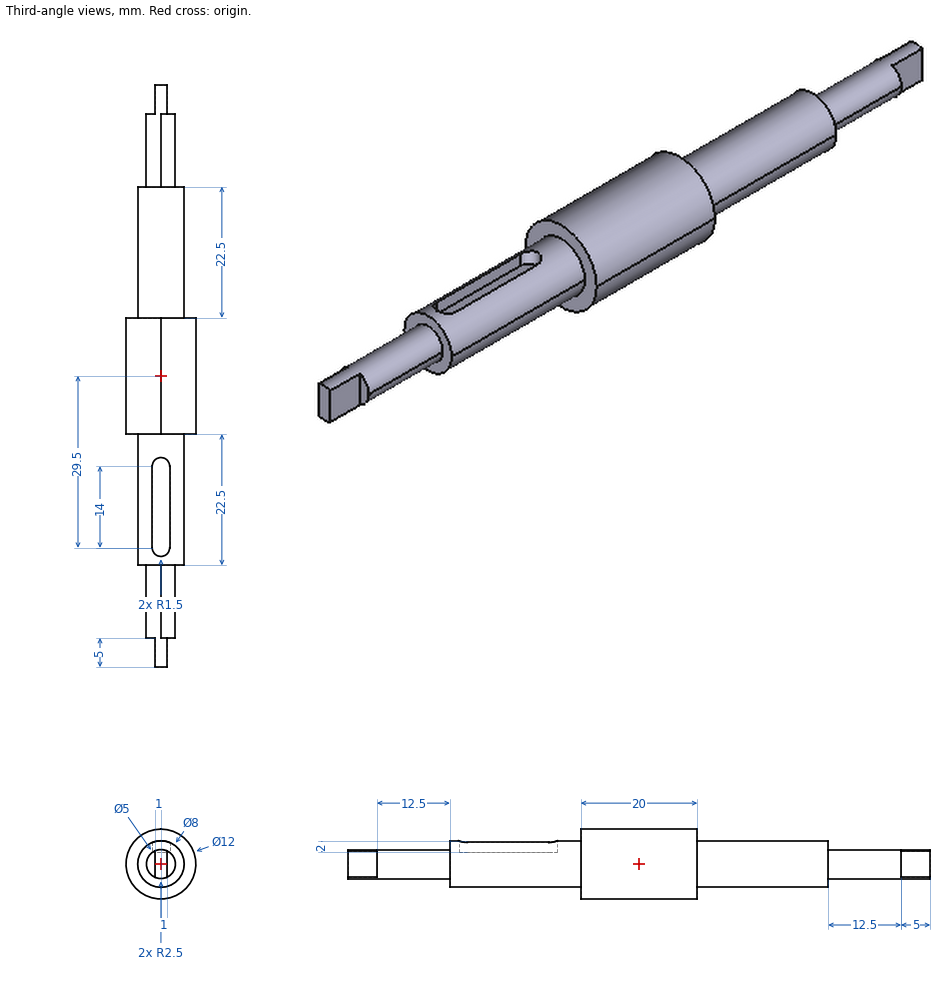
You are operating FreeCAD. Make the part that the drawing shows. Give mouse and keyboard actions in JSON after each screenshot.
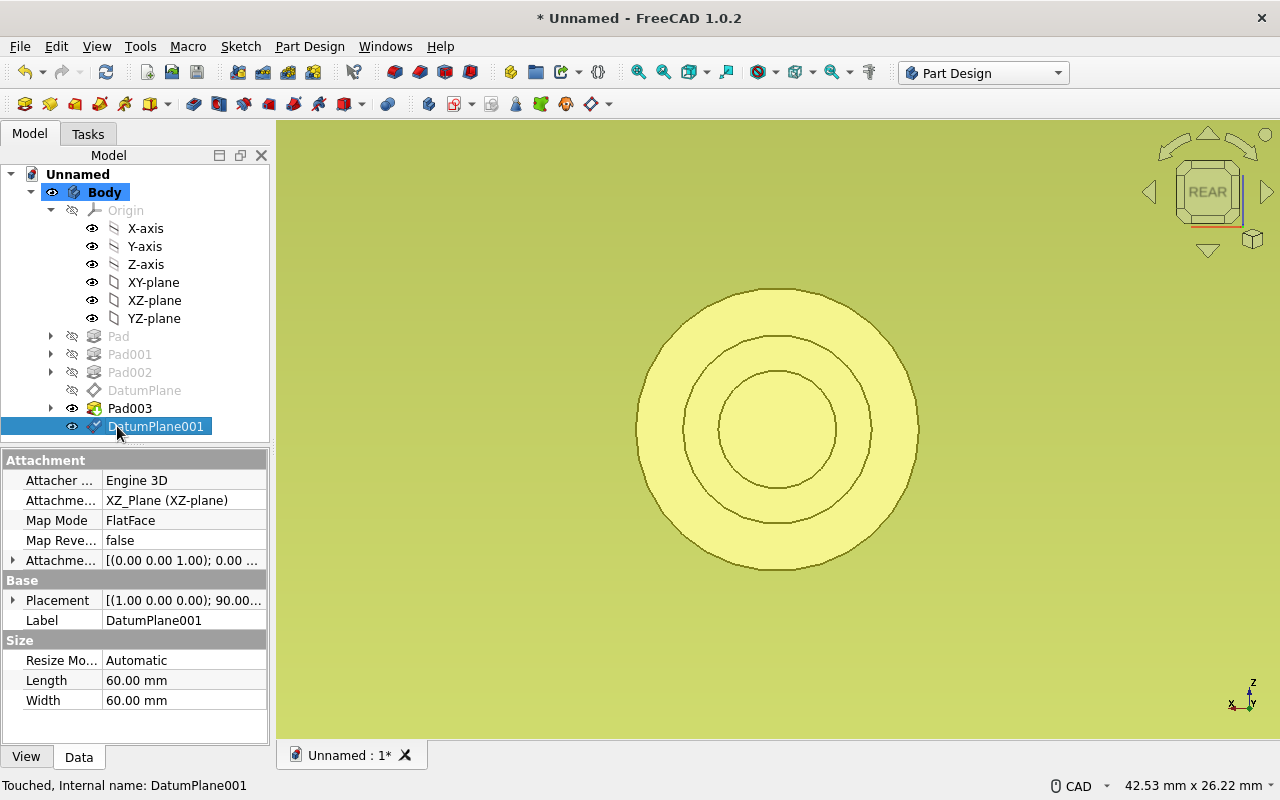
{"action": "left_click", "coordinate": [454, 104]}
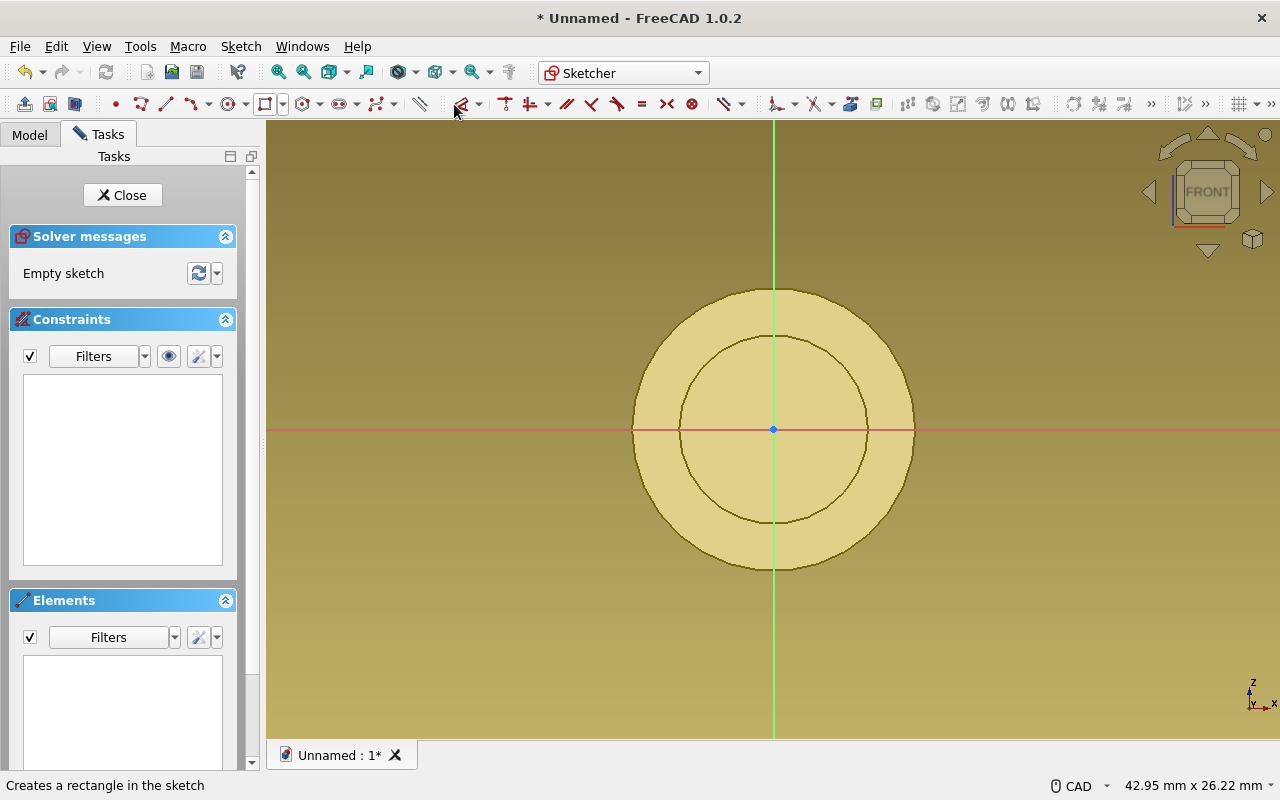
{"action": "scroll", "coordinate": [803, 429], "scroll_direction": "up", "scroll_amount": 6}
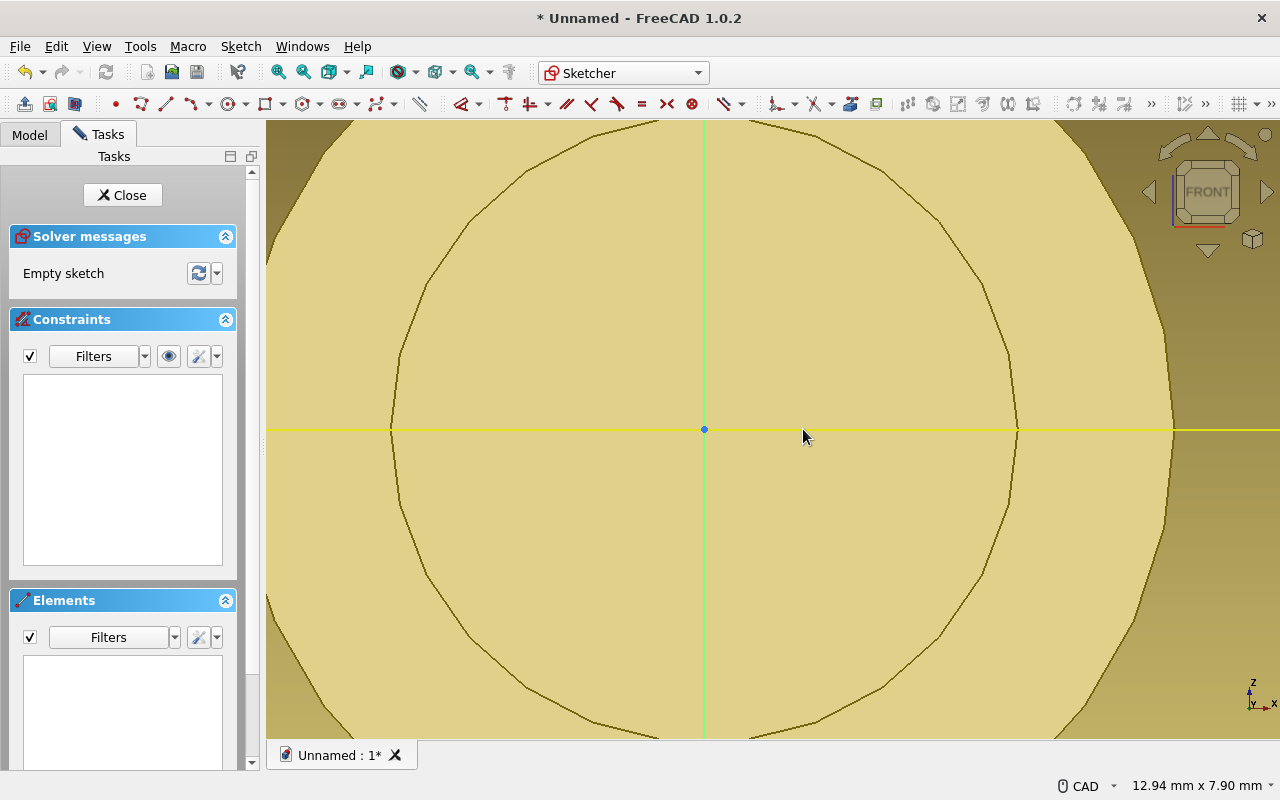
{"action": "key", "text": "g c"}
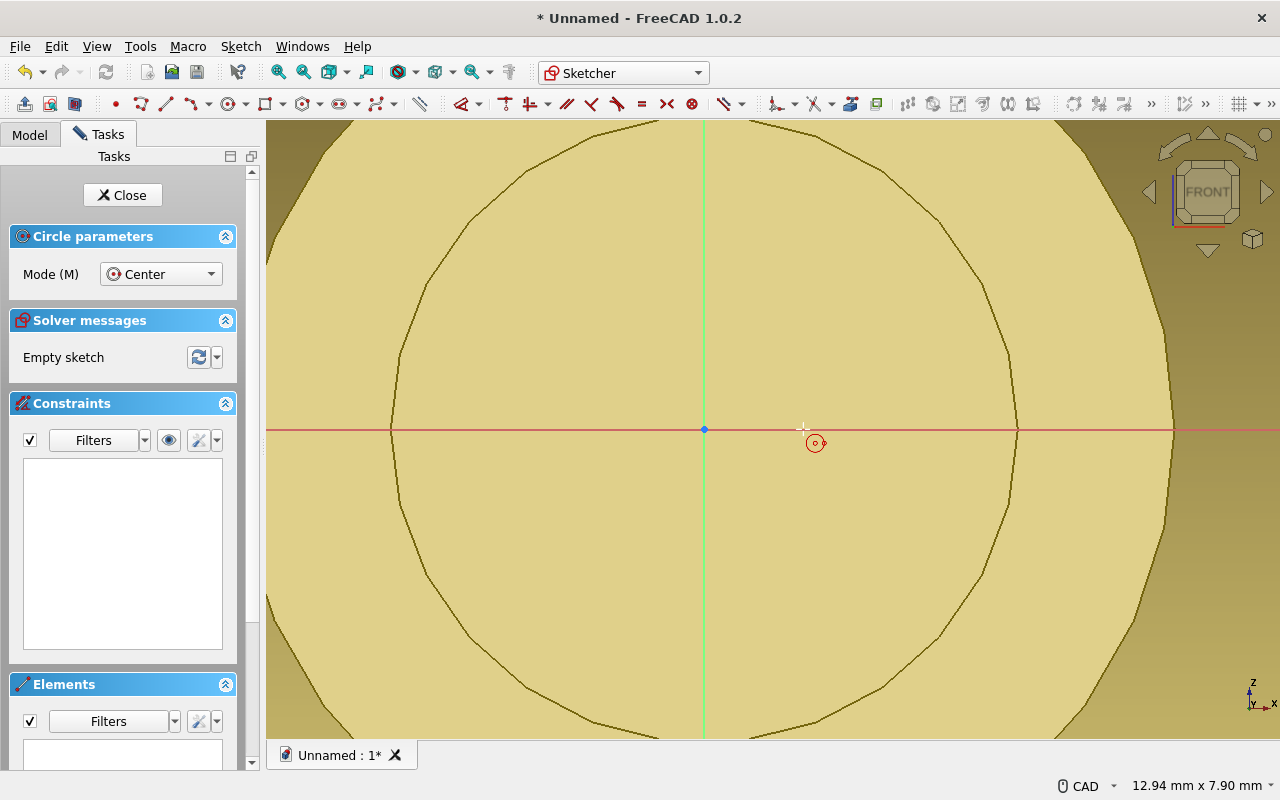
{"action": "left_click", "coordinate": [704, 429]}
{"action": "mouse_move", "coordinate": [843, 291]}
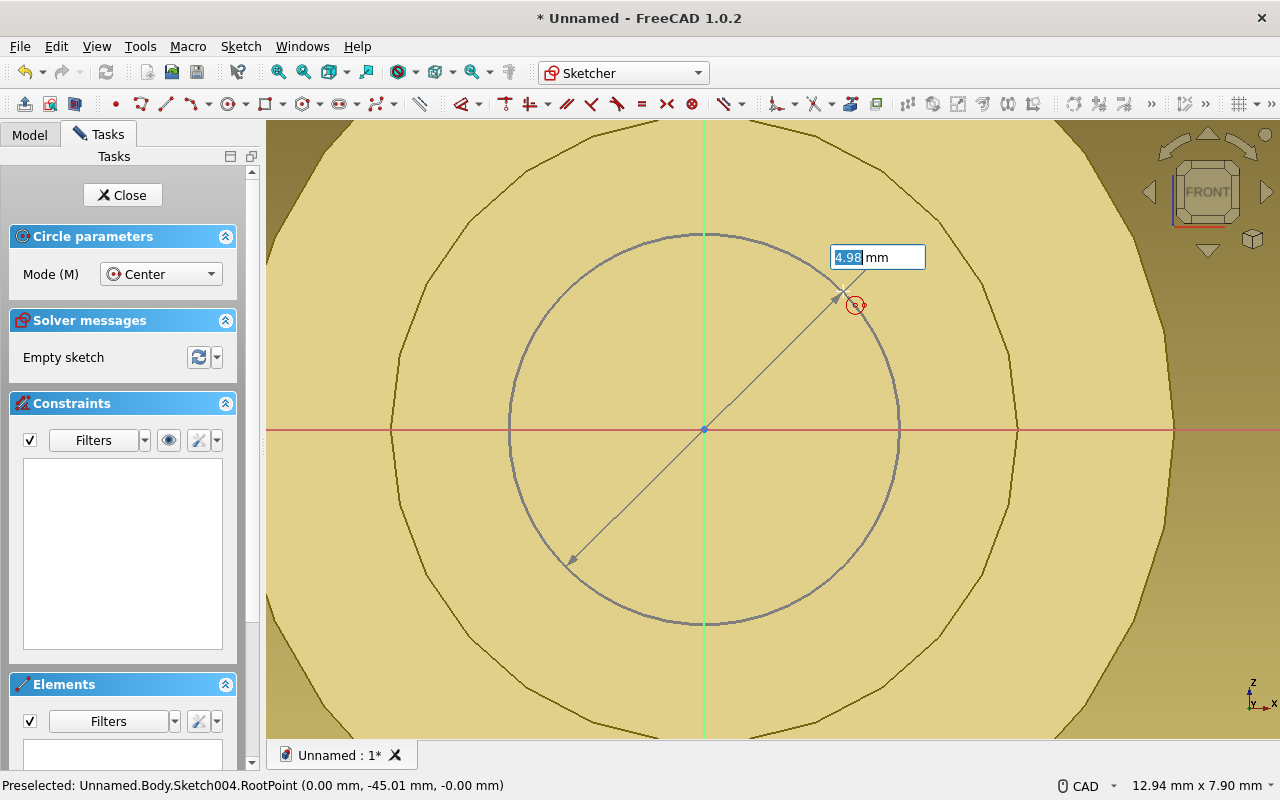
{"action": "type", "text": "5"}
{"action": "key", "text": "Return"}
{"action": "key", "text": "Escape"}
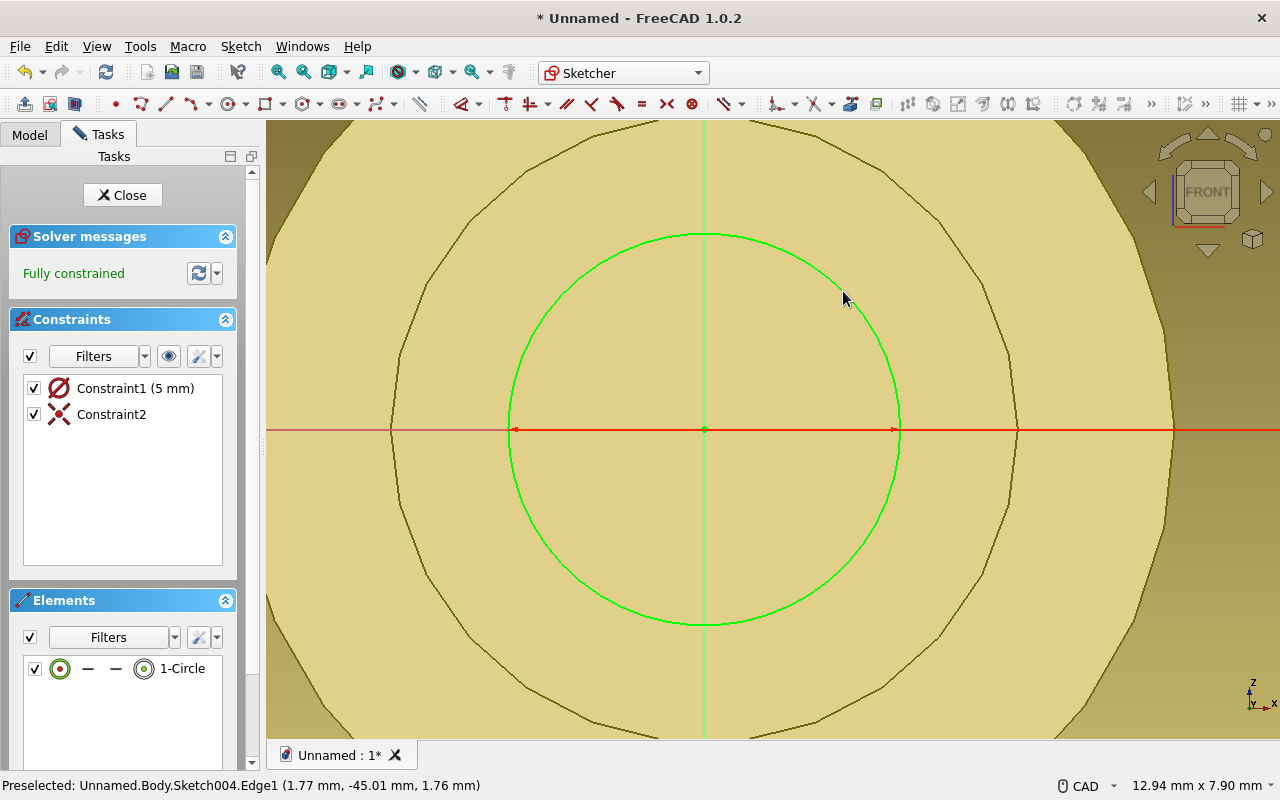
{"action": "left_click", "coordinate": [123, 195]}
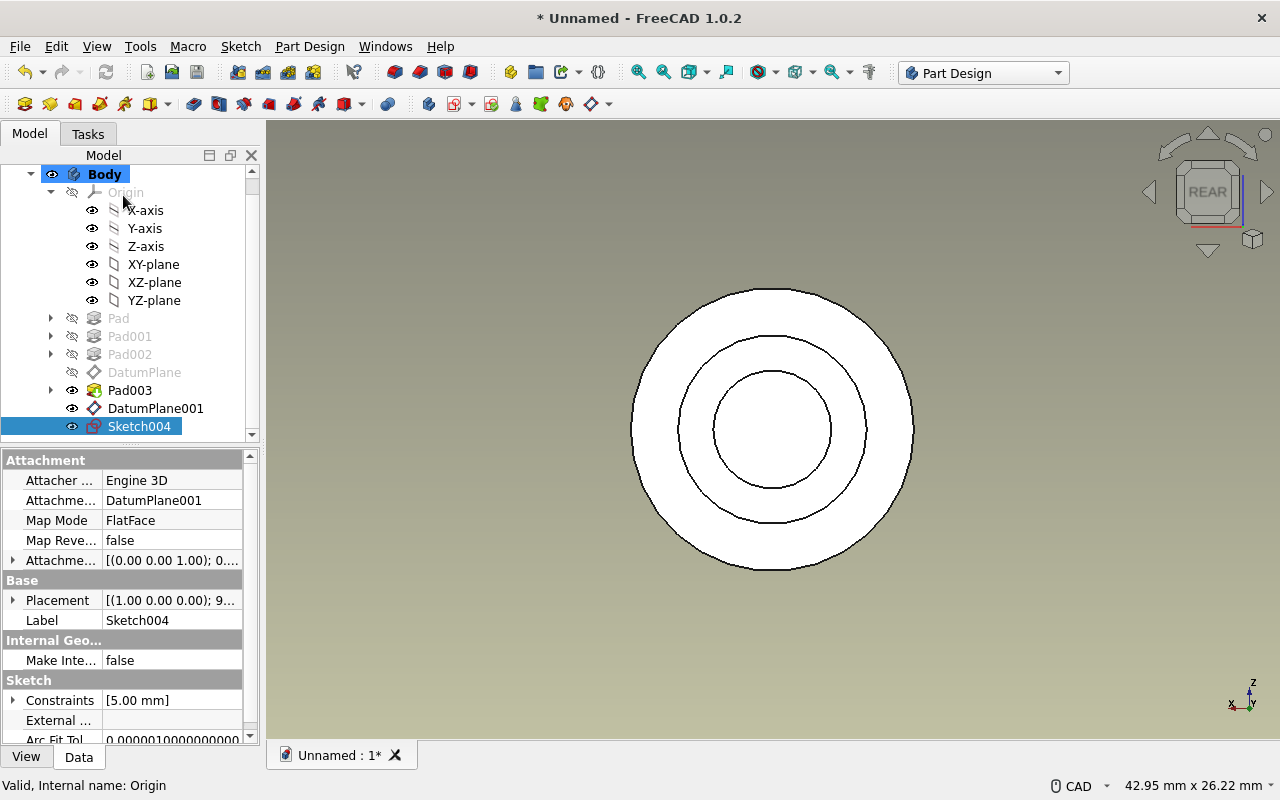
{"action": "left_click", "coordinate": [25, 104]}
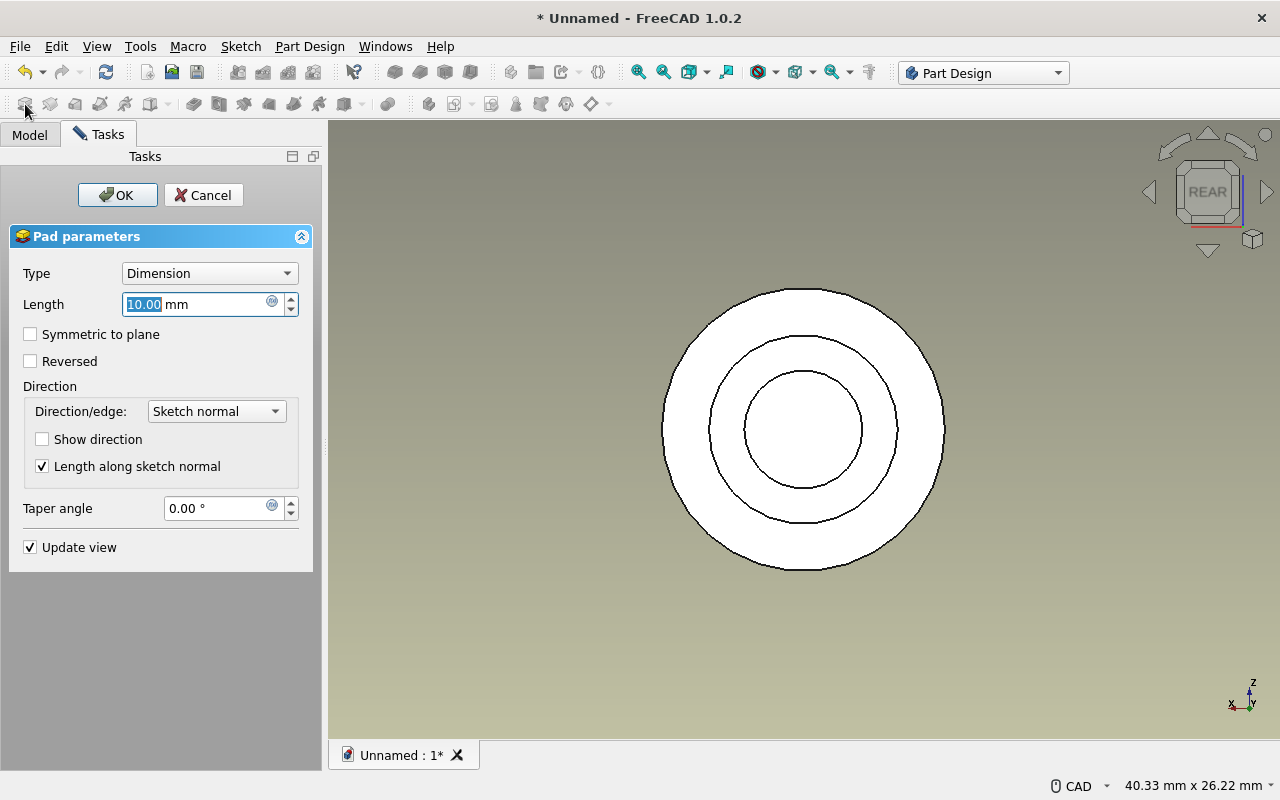
{"action": "type", "text": "12.5"}
{"action": "key", "text": "Tab"}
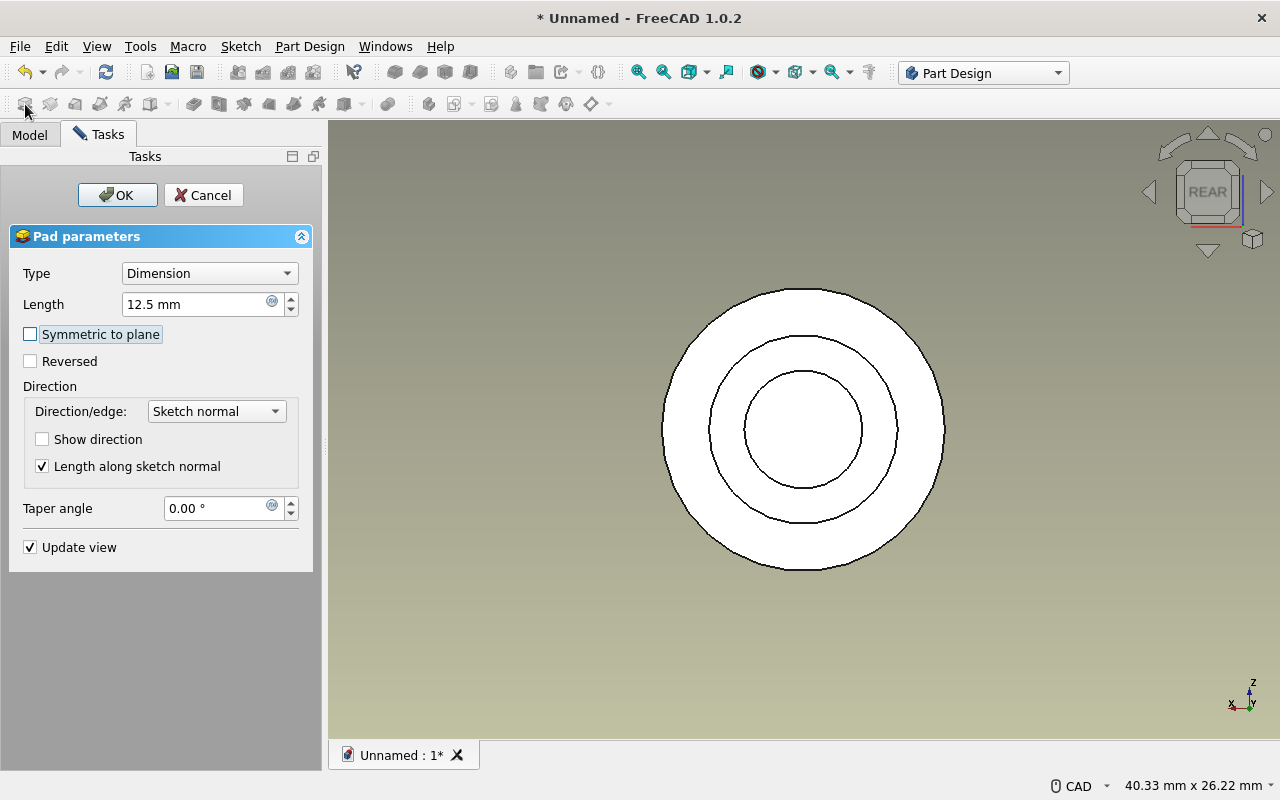
{"action": "left_click", "coordinate": [31, 361]}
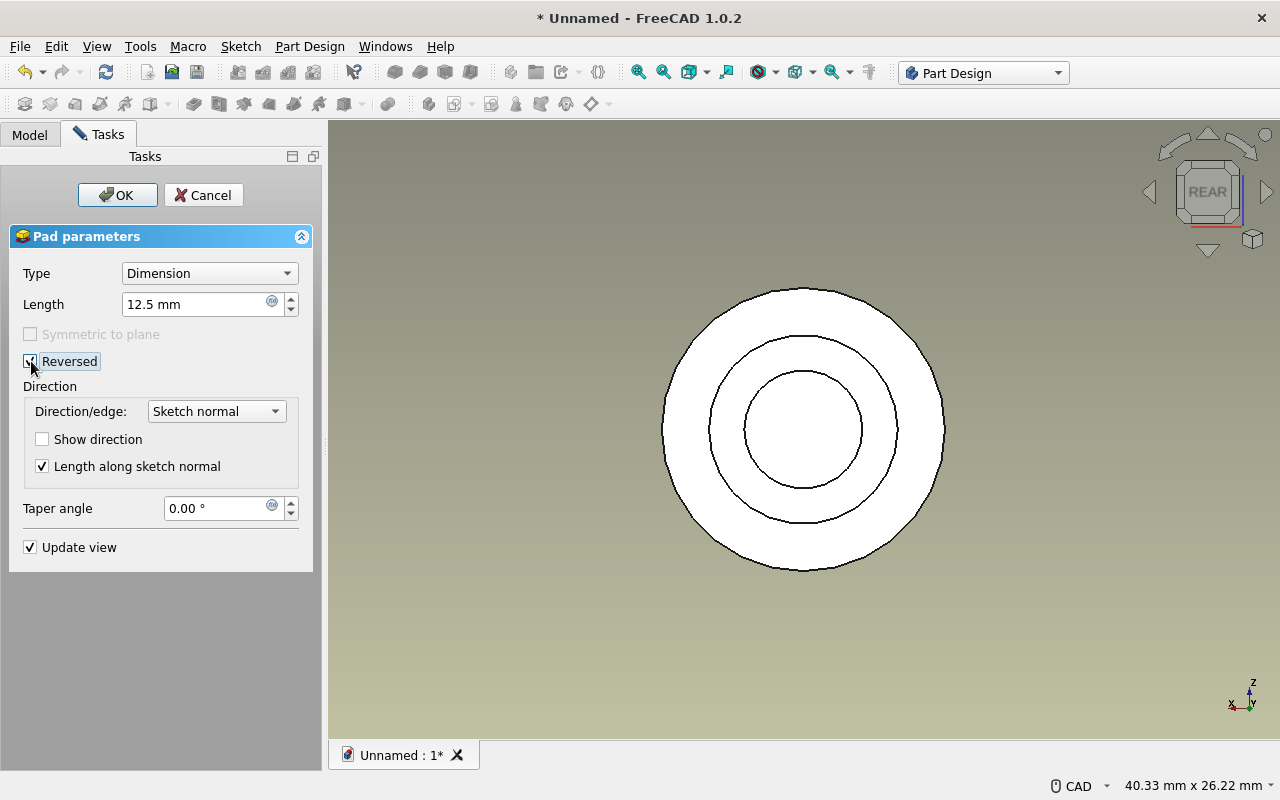
{"action": "left_click", "coordinate": [118, 195]}